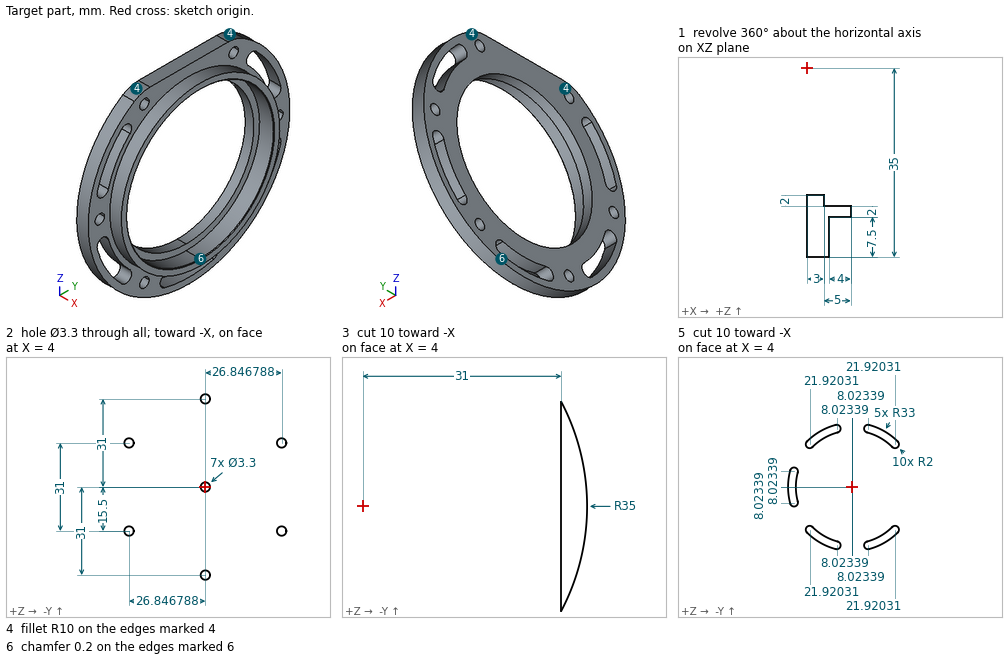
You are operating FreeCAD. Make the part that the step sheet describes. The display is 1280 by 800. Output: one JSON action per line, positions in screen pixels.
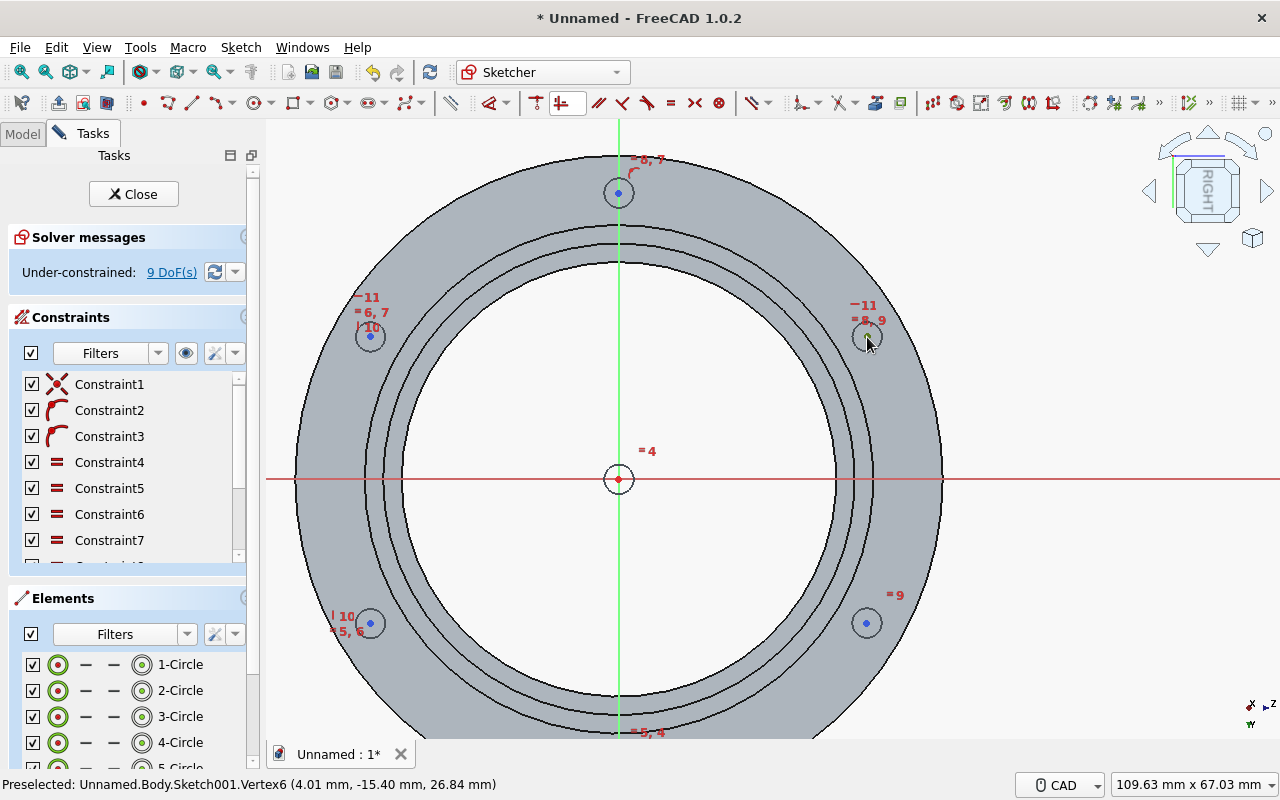
{"action": "left_click", "coordinate": [867, 623]}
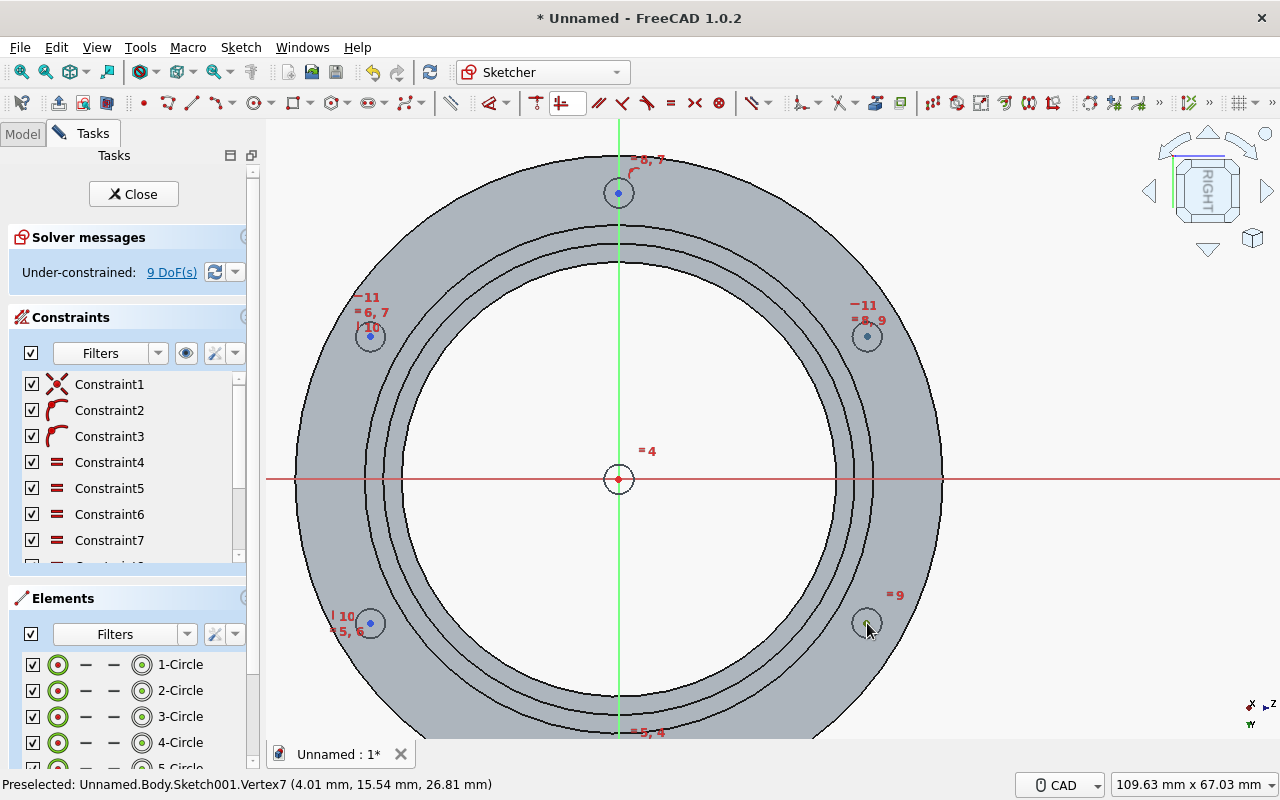
{"action": "key", "text": "v"}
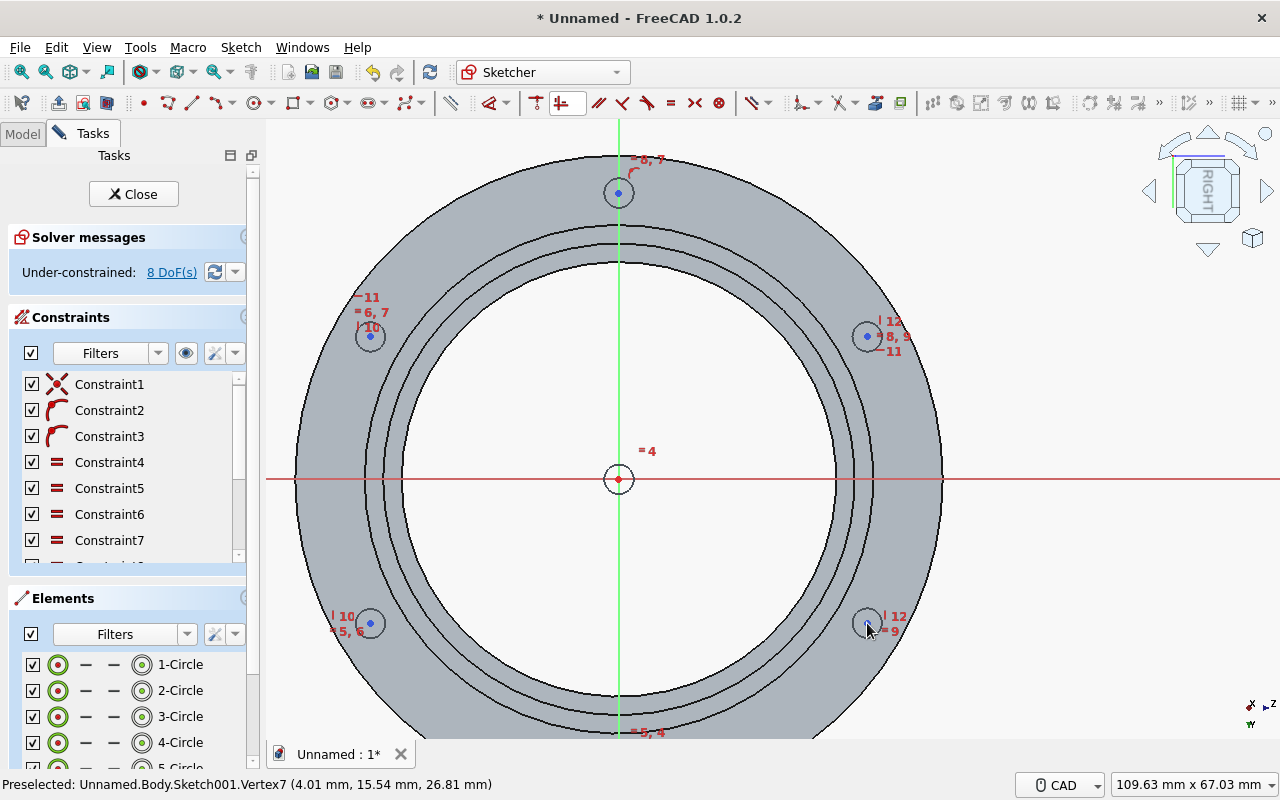
{"action": "left_click", "coordinate": [371, 624]}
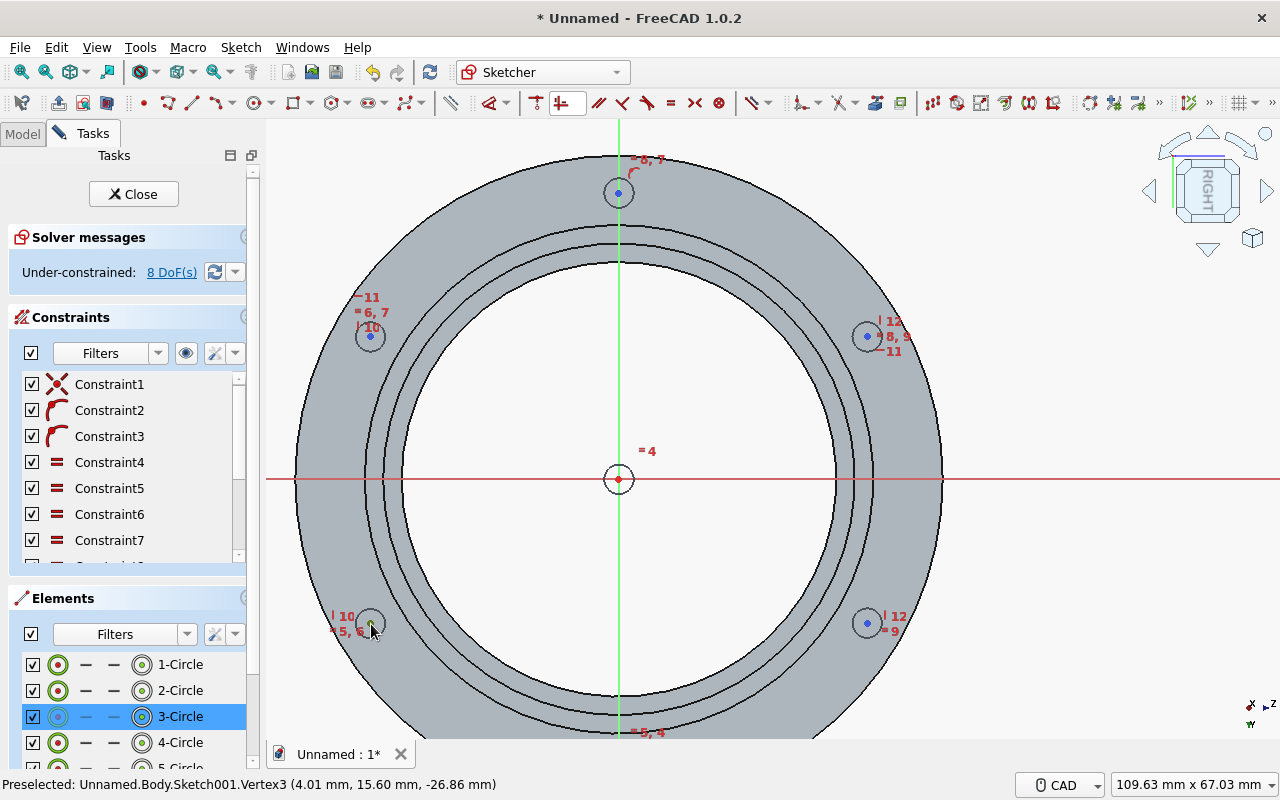
{"action": "left_click", "coordinate": [867, 623]}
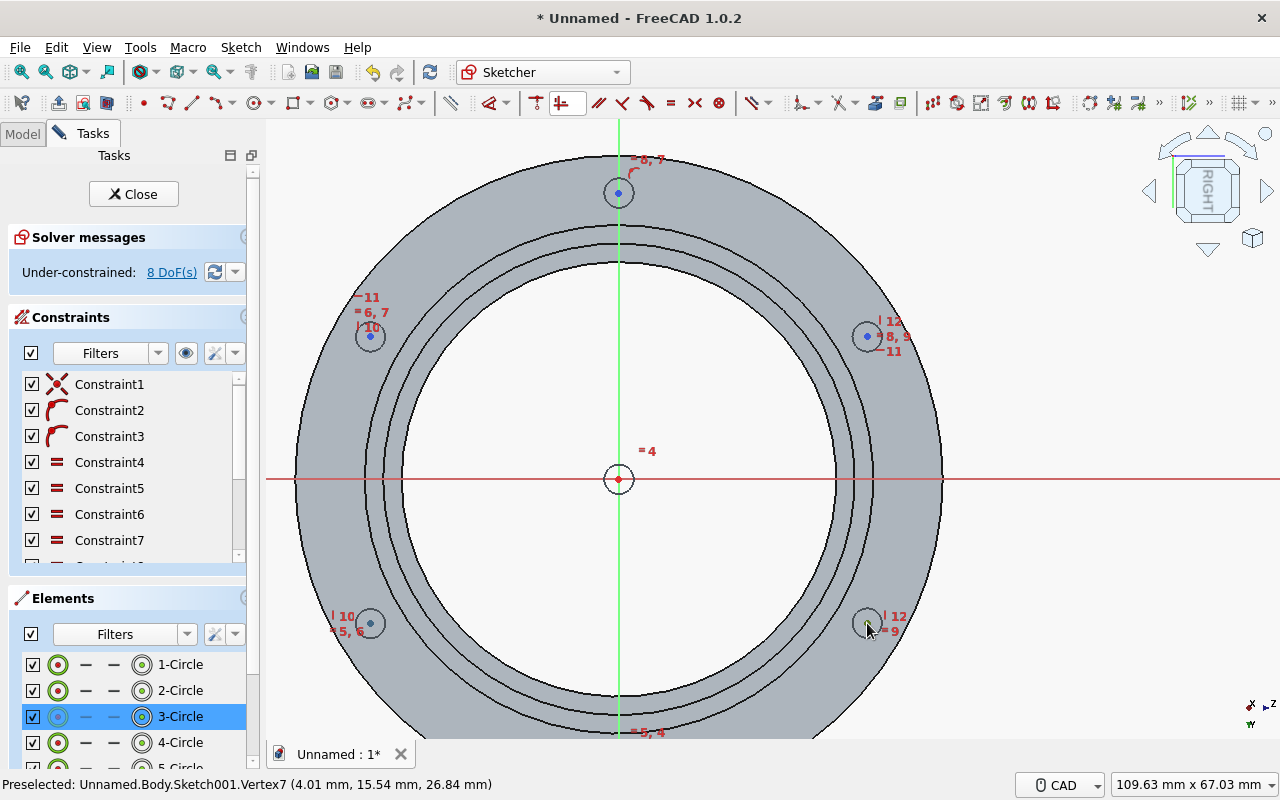
{"action": "key", "text": "h"}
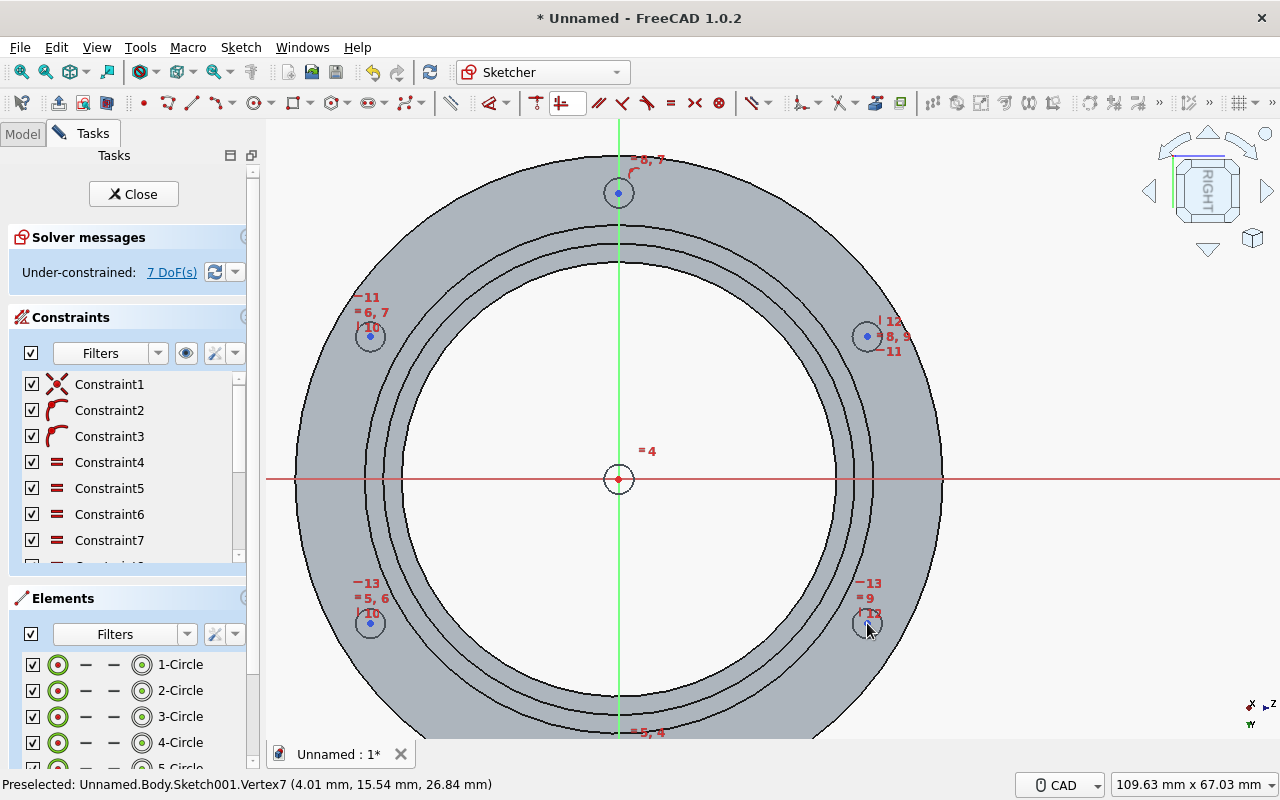
{"action": "left_click", "coordinate": [490, 104]}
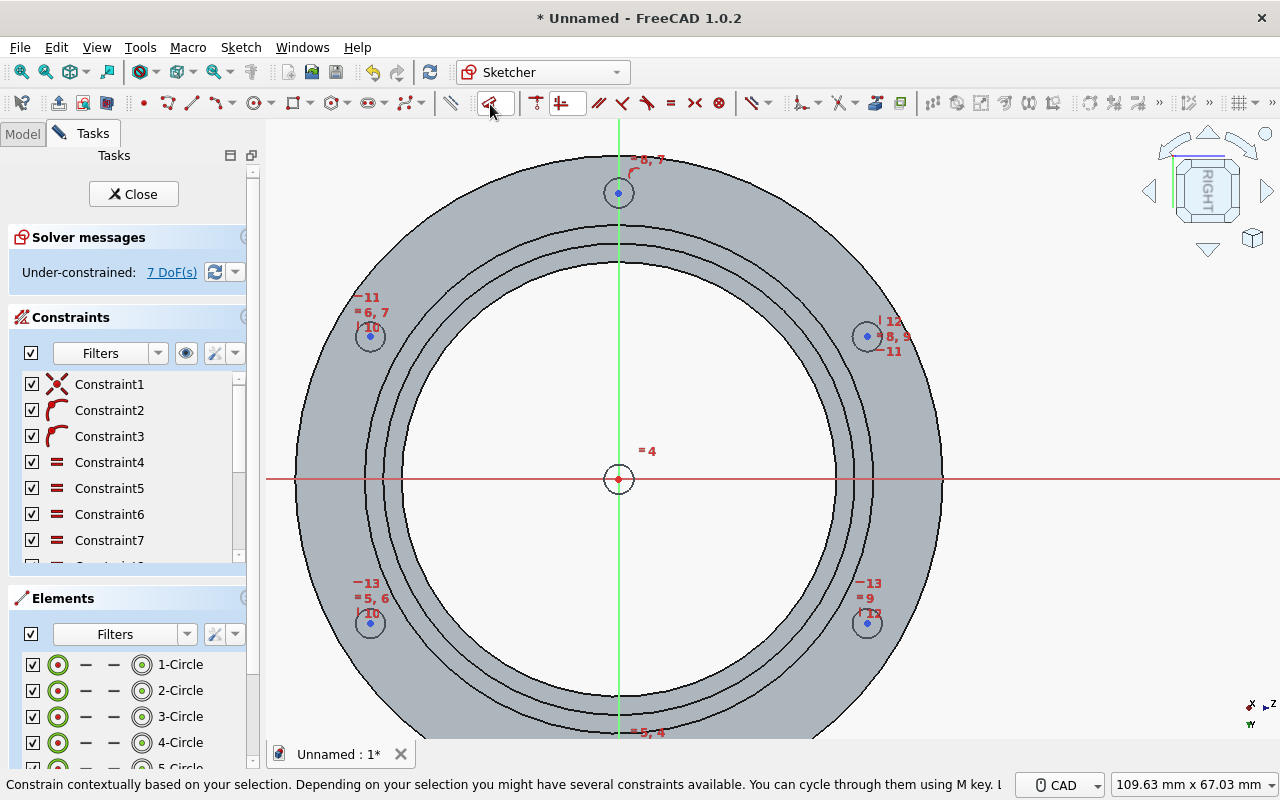
{"action": "scroll", "coordinate": [629, 469], "scroll_direction": "up", "scroll_amount": 2}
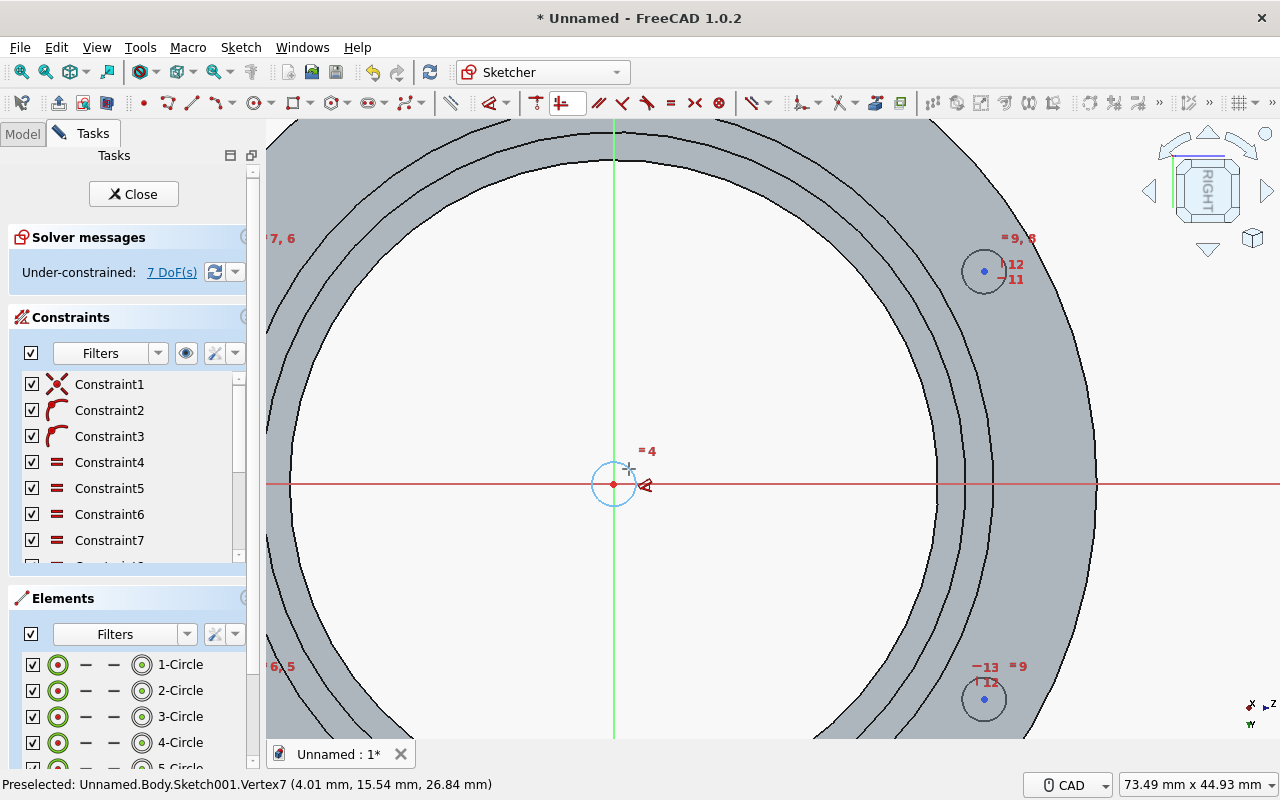
{"action": "left_click", "coordinate": [629, 469]}
{"action": "left_click", "coordinate": [652, 446]}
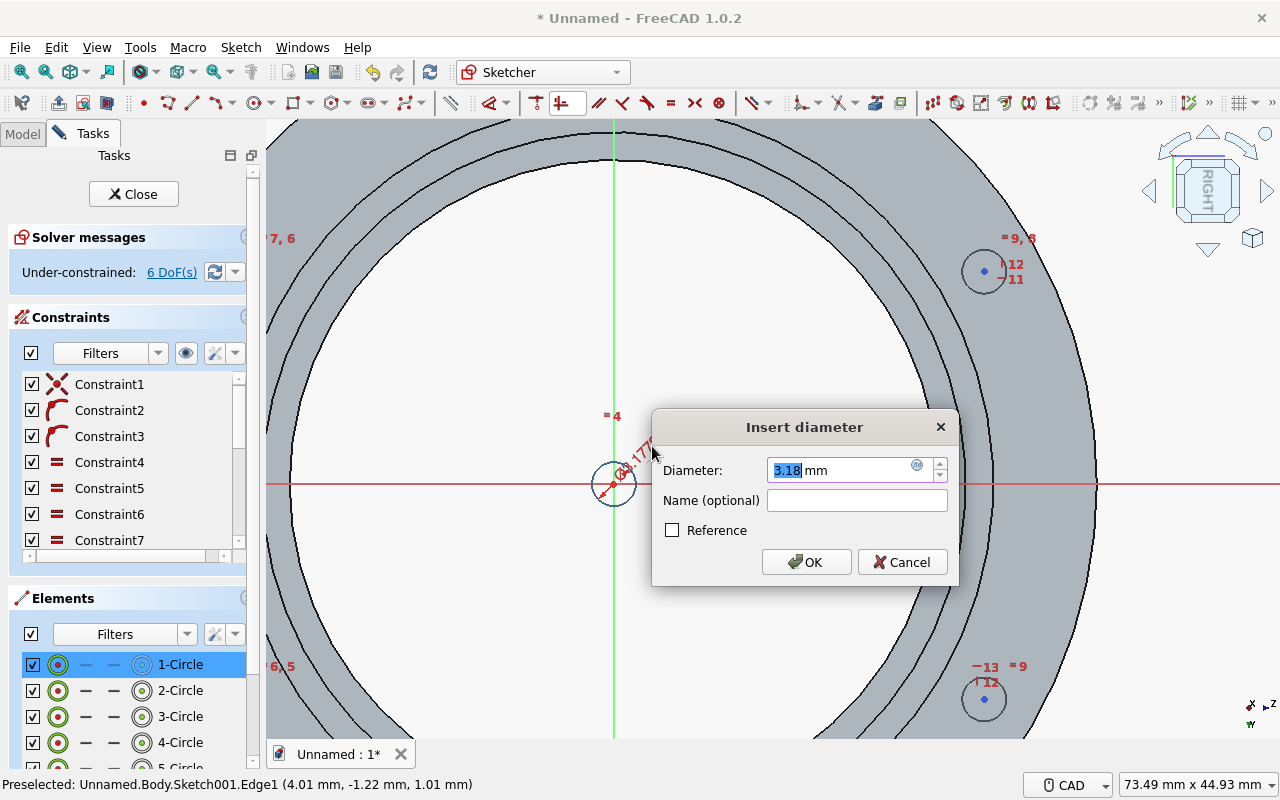
{"action": "type", "text": "3.3"}
{"action": "key", "text": "Return"}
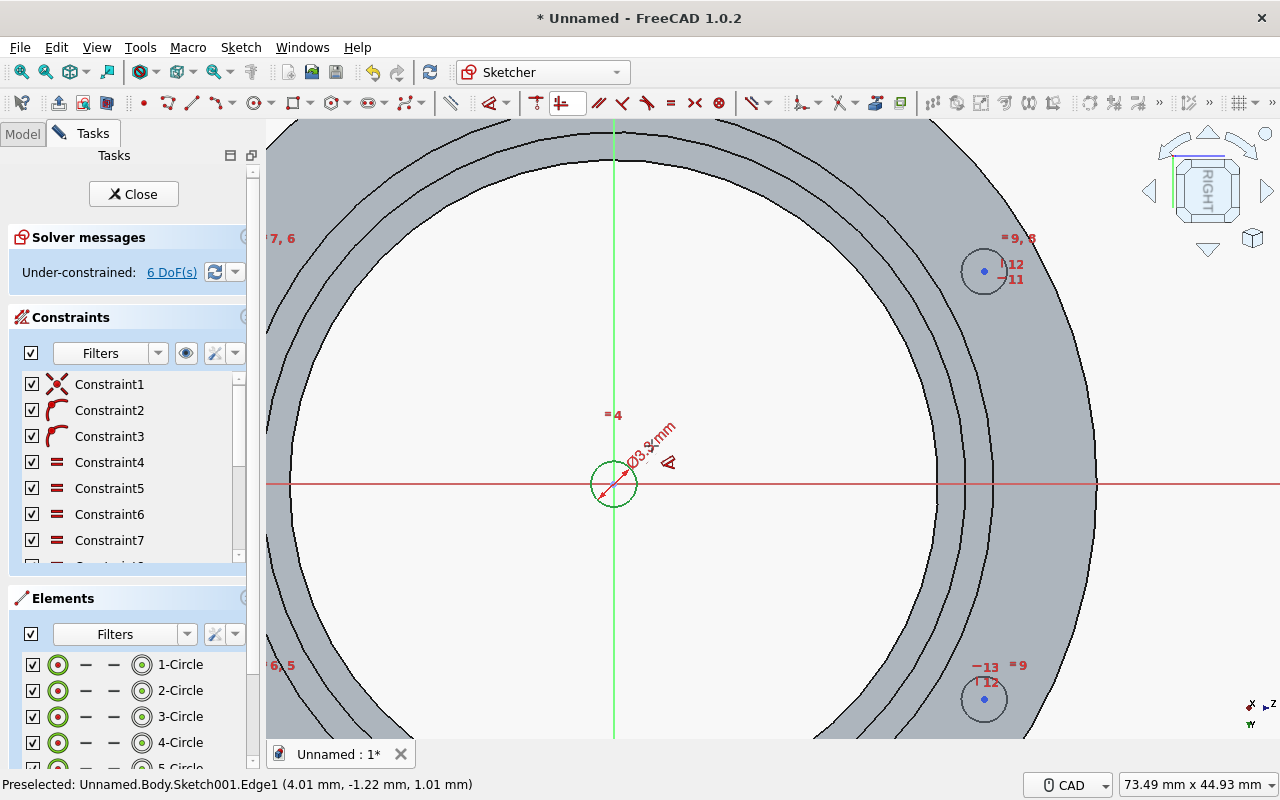
{"action": "scroll", "coordinate": [778, 384], "scroll_direction": "down", "scroll_amount": 4}